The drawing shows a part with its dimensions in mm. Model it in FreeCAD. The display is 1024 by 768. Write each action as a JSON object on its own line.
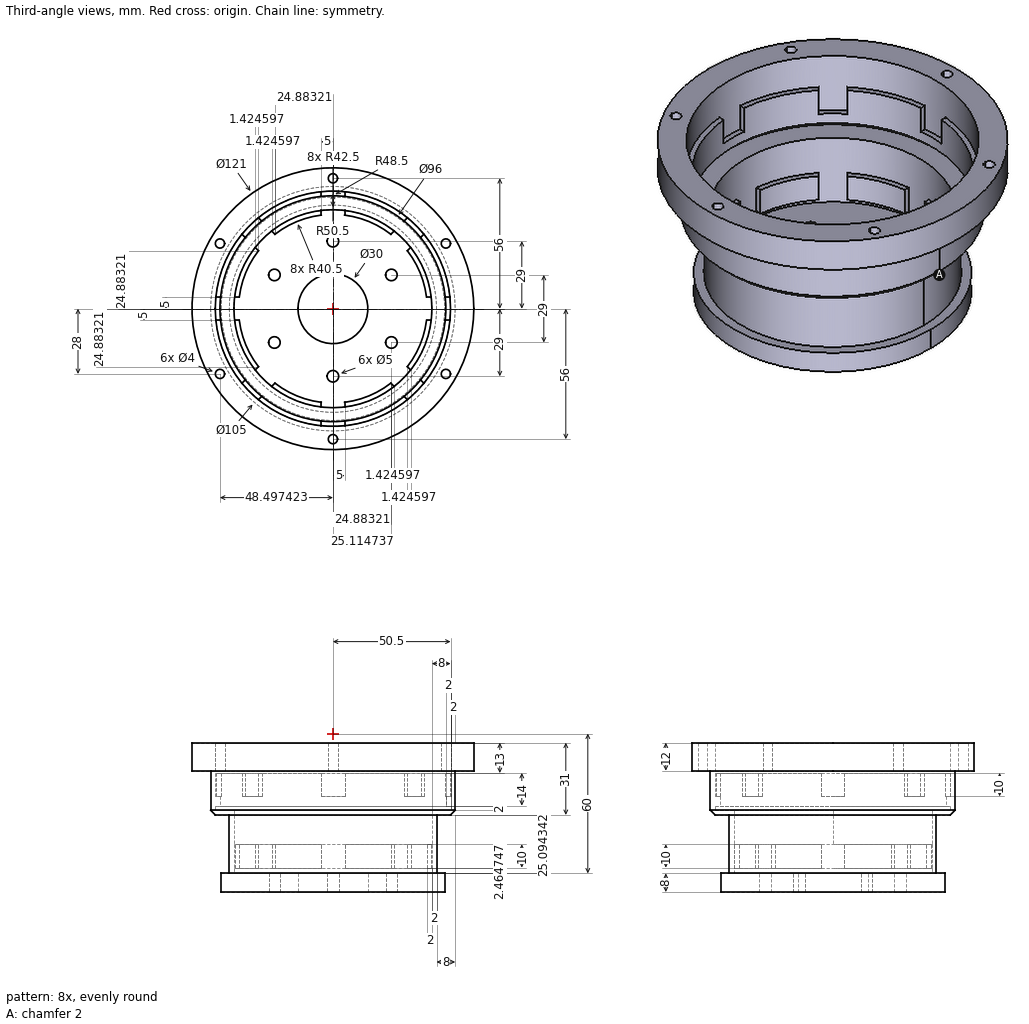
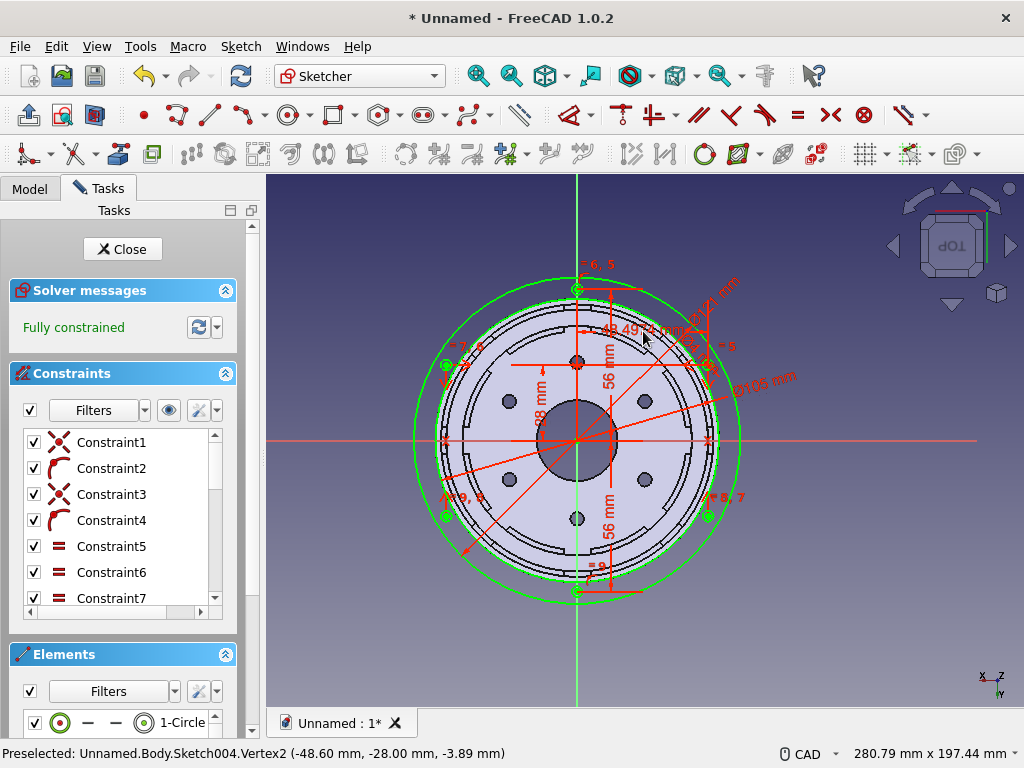
{"action": "left_click", "coordinate": [123, 249]}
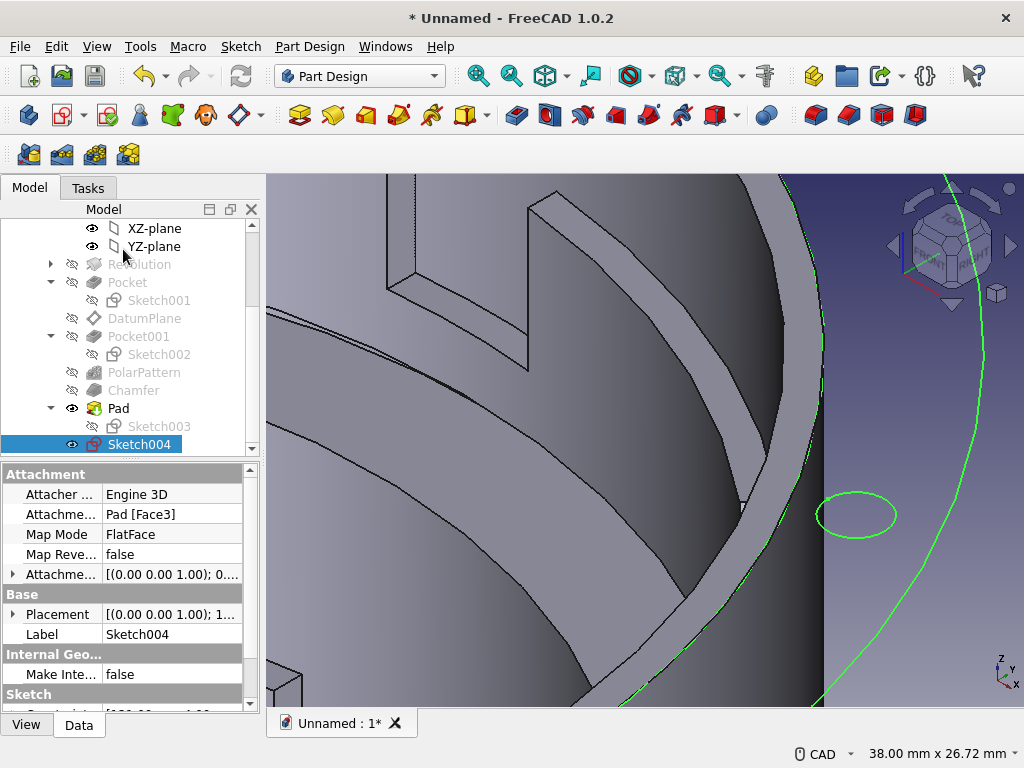
{"action": "left_click", "coordinate": [300, 116]}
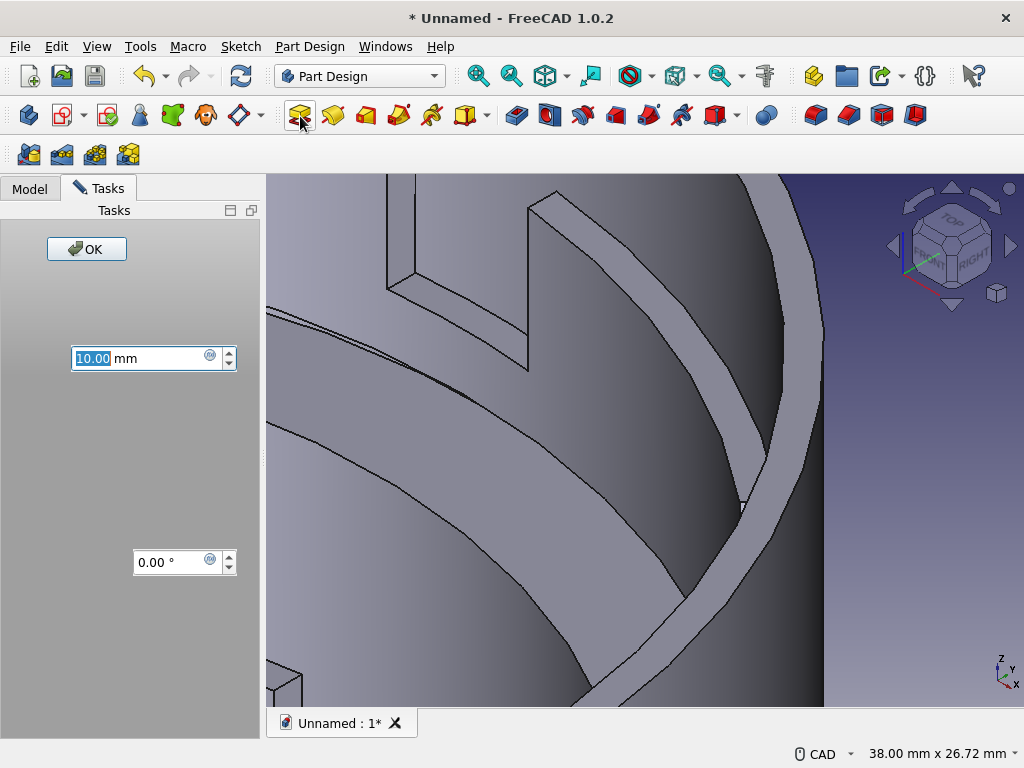
{"action": "type", "text": "12"}
{"action": "key", "text": "Tab"}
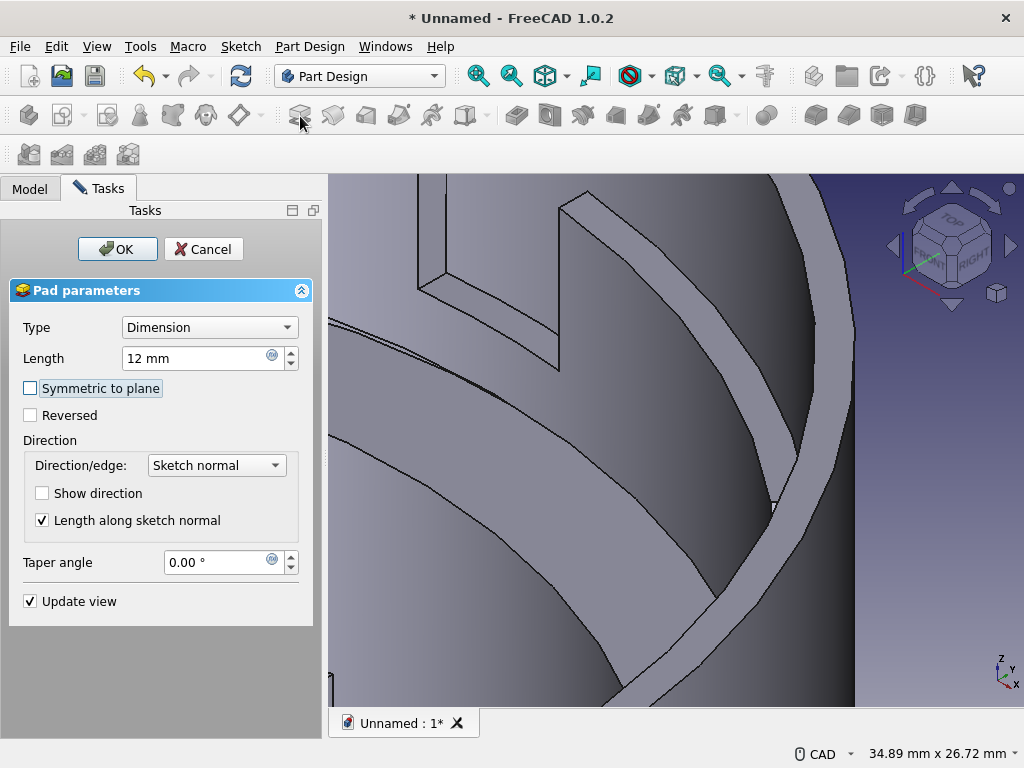
{"action": "left_click", "coordinate": [31, 415]}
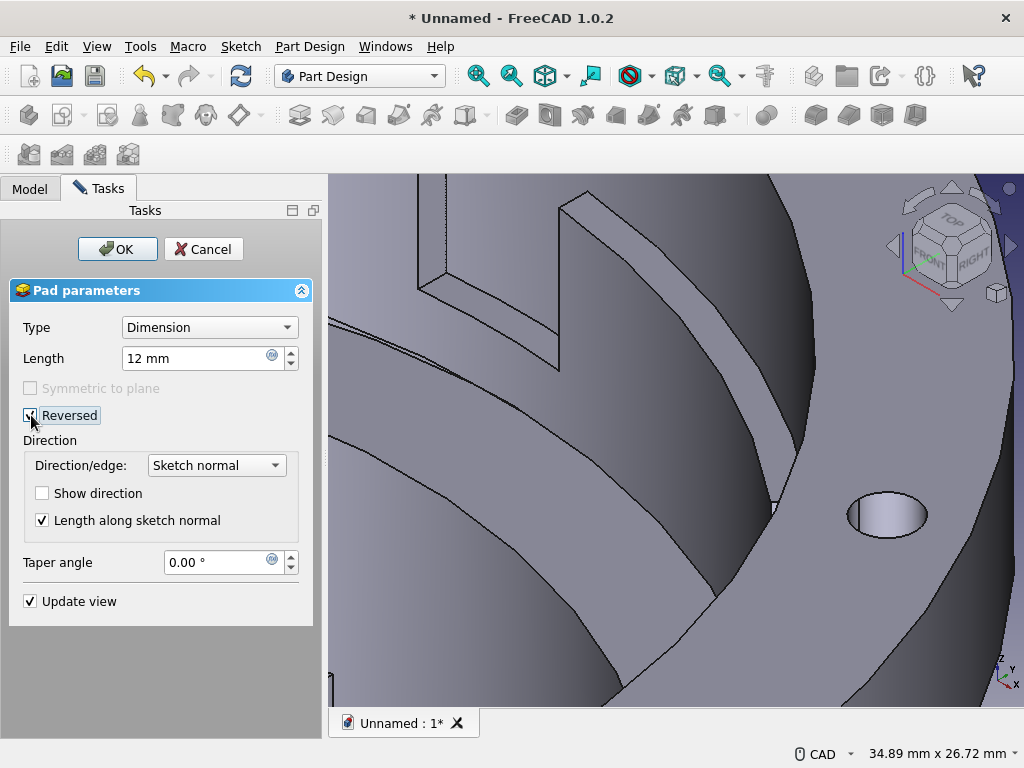
{"action": "left_click", "coordinate": [118, 249]}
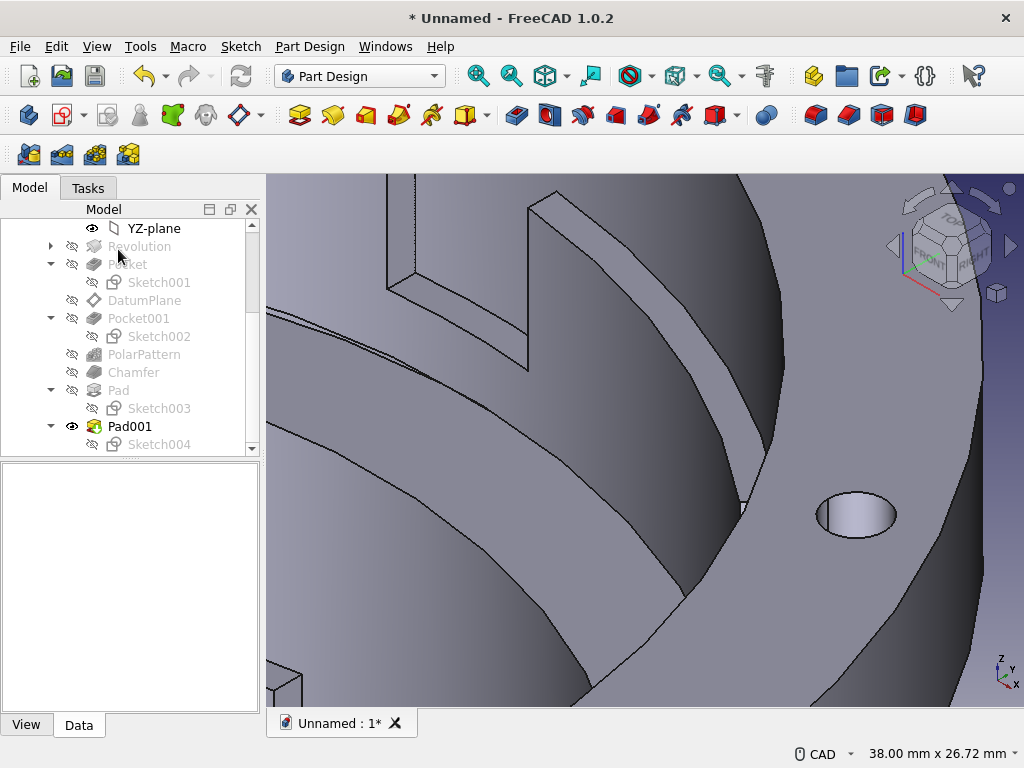
{"action": "left_click", "coordinate": [479, 76]}